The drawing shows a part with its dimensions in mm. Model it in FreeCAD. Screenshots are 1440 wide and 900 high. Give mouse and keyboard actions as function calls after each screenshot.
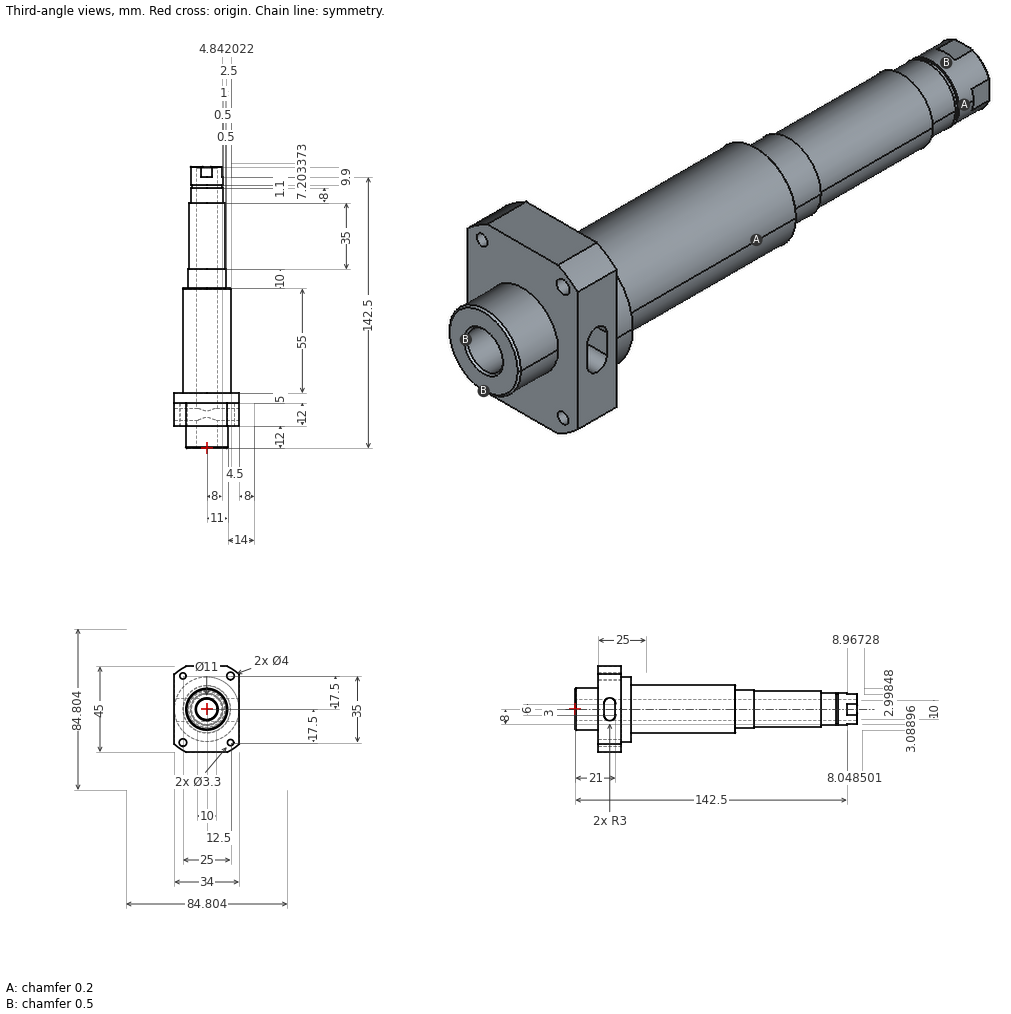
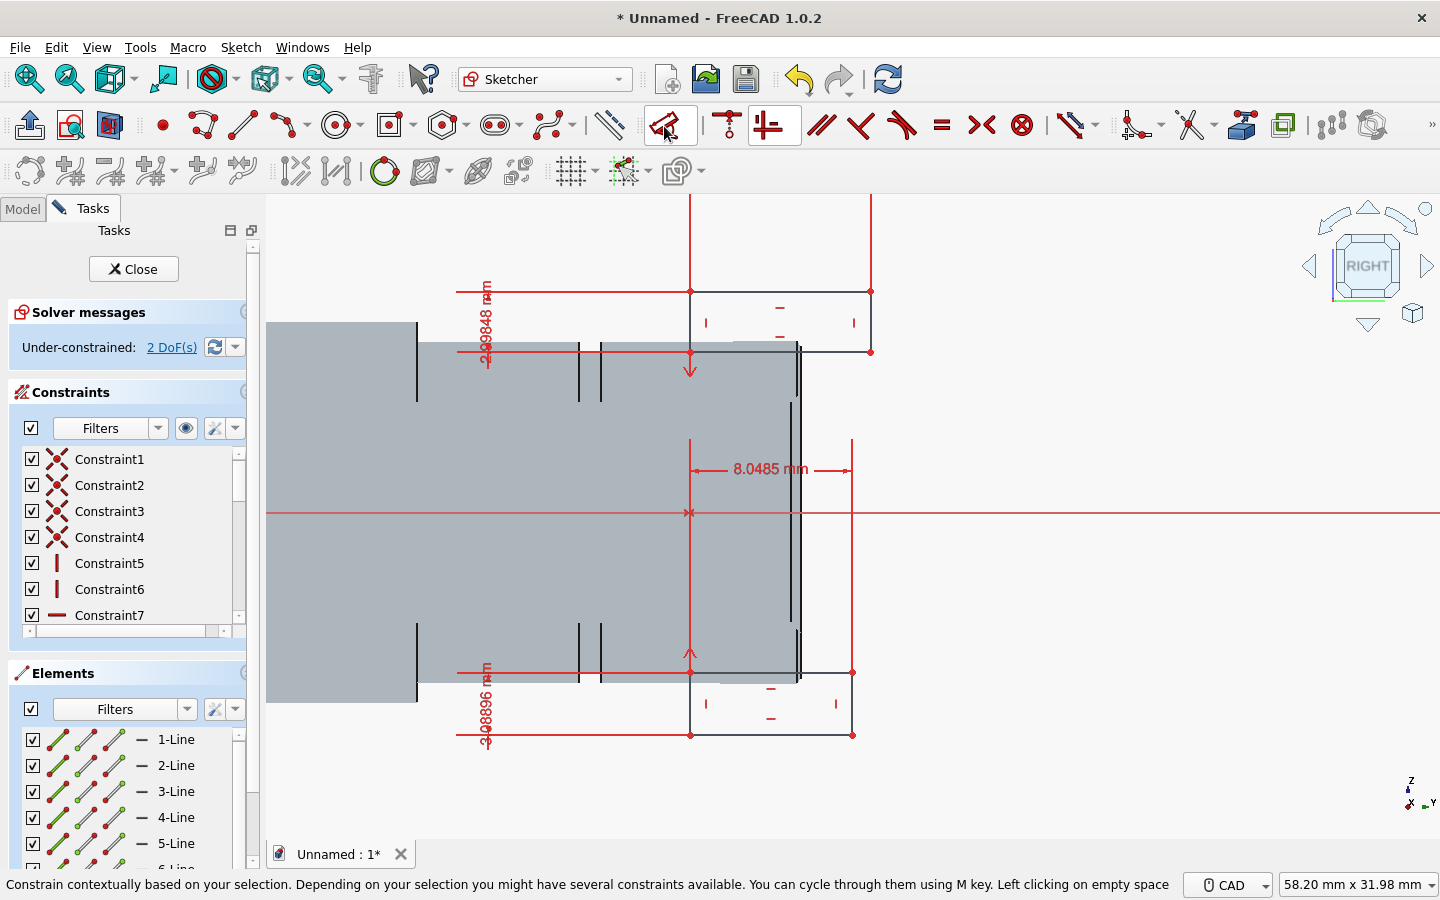
click(690, 673)
click(724, 593)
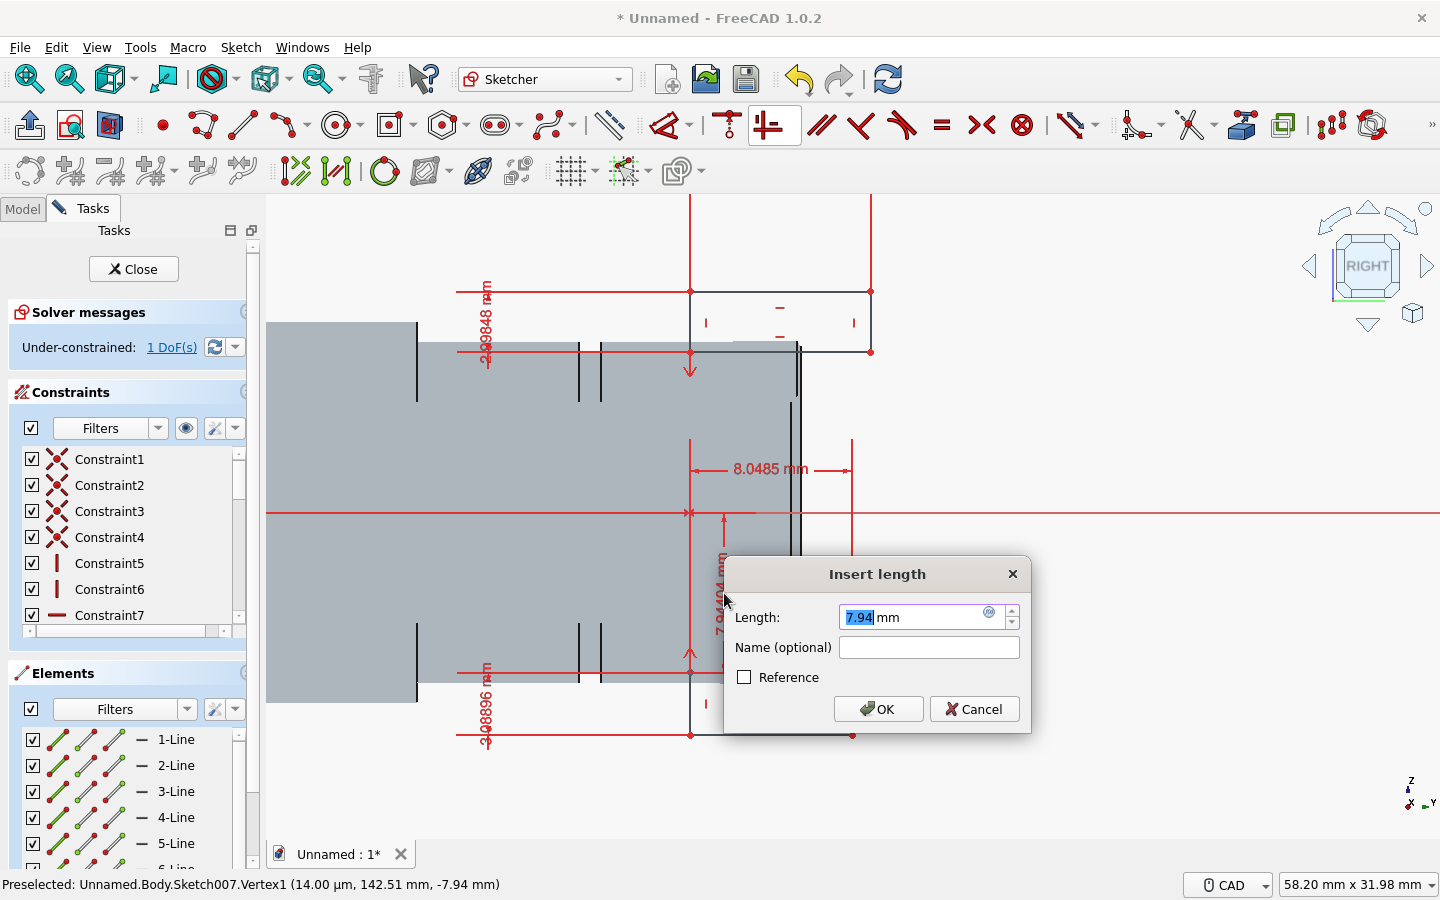
text(8)
key(Return)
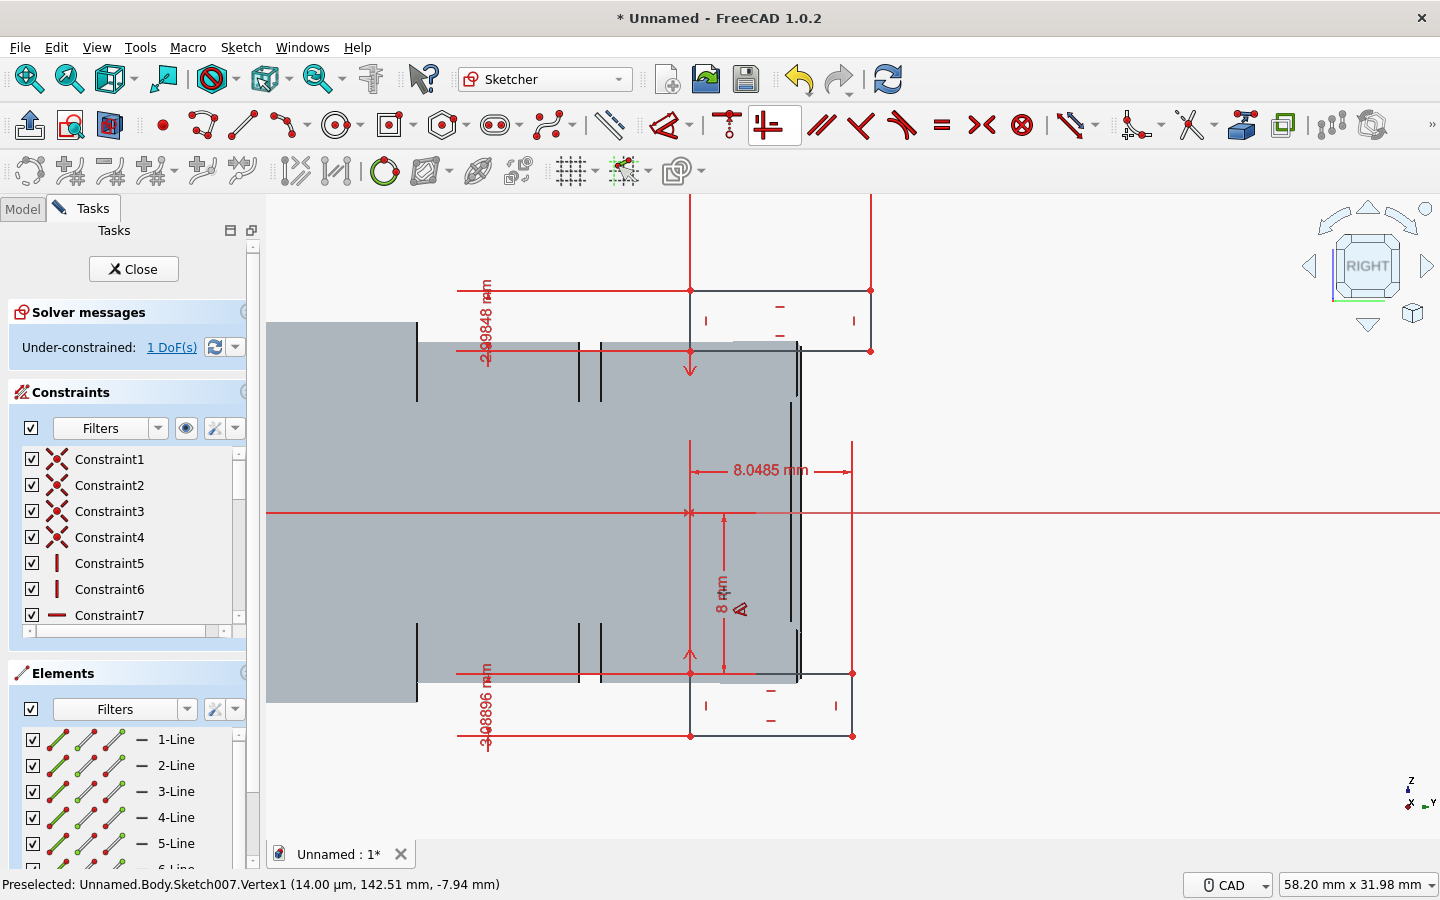
click(690, 674)
click(492, 708)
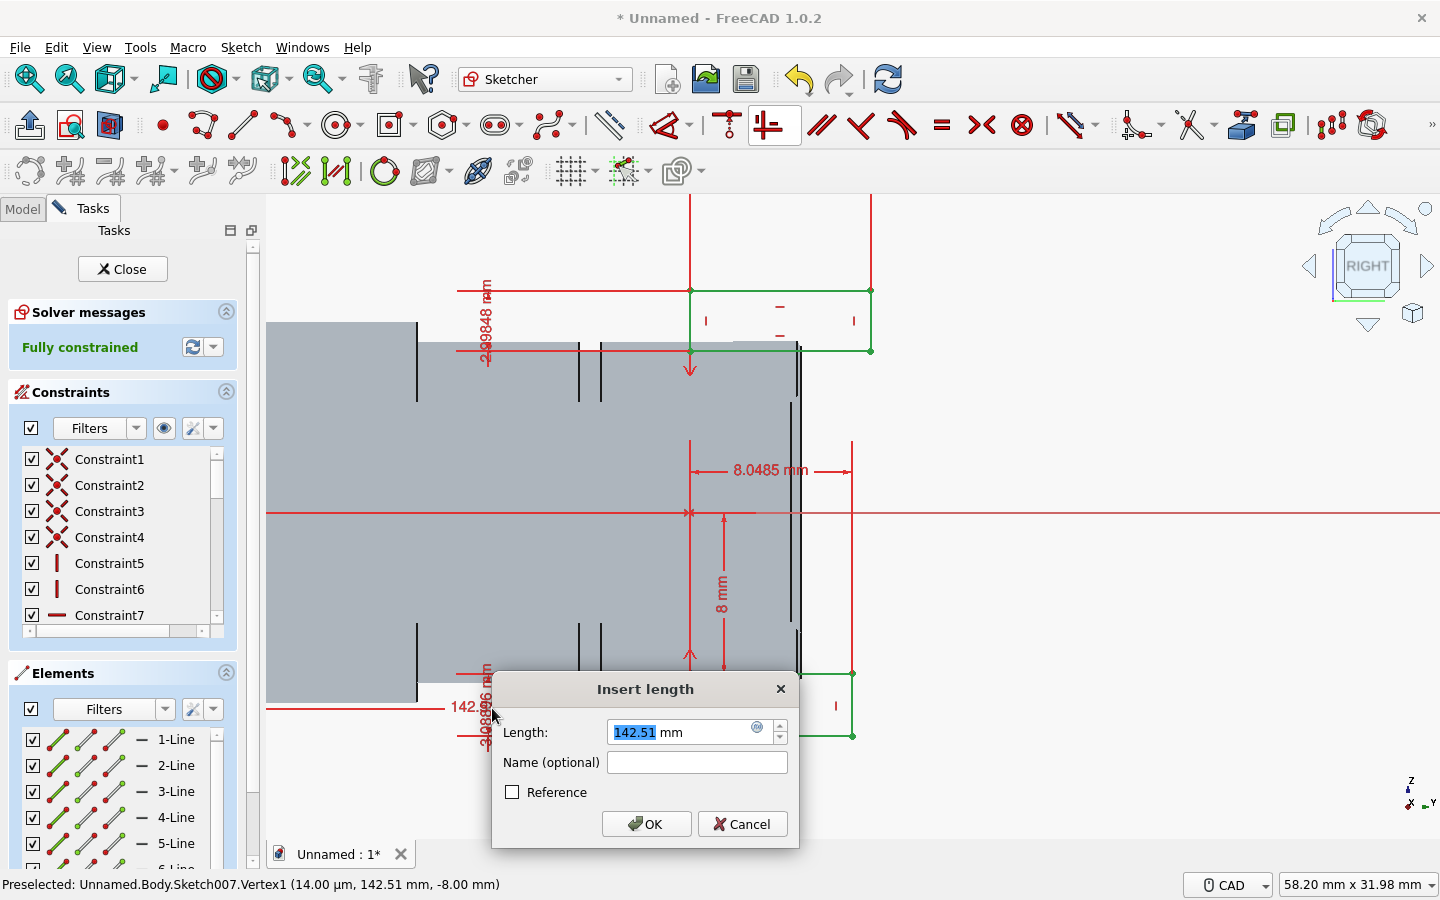
text(142.5)
key(Return)
key(Escape)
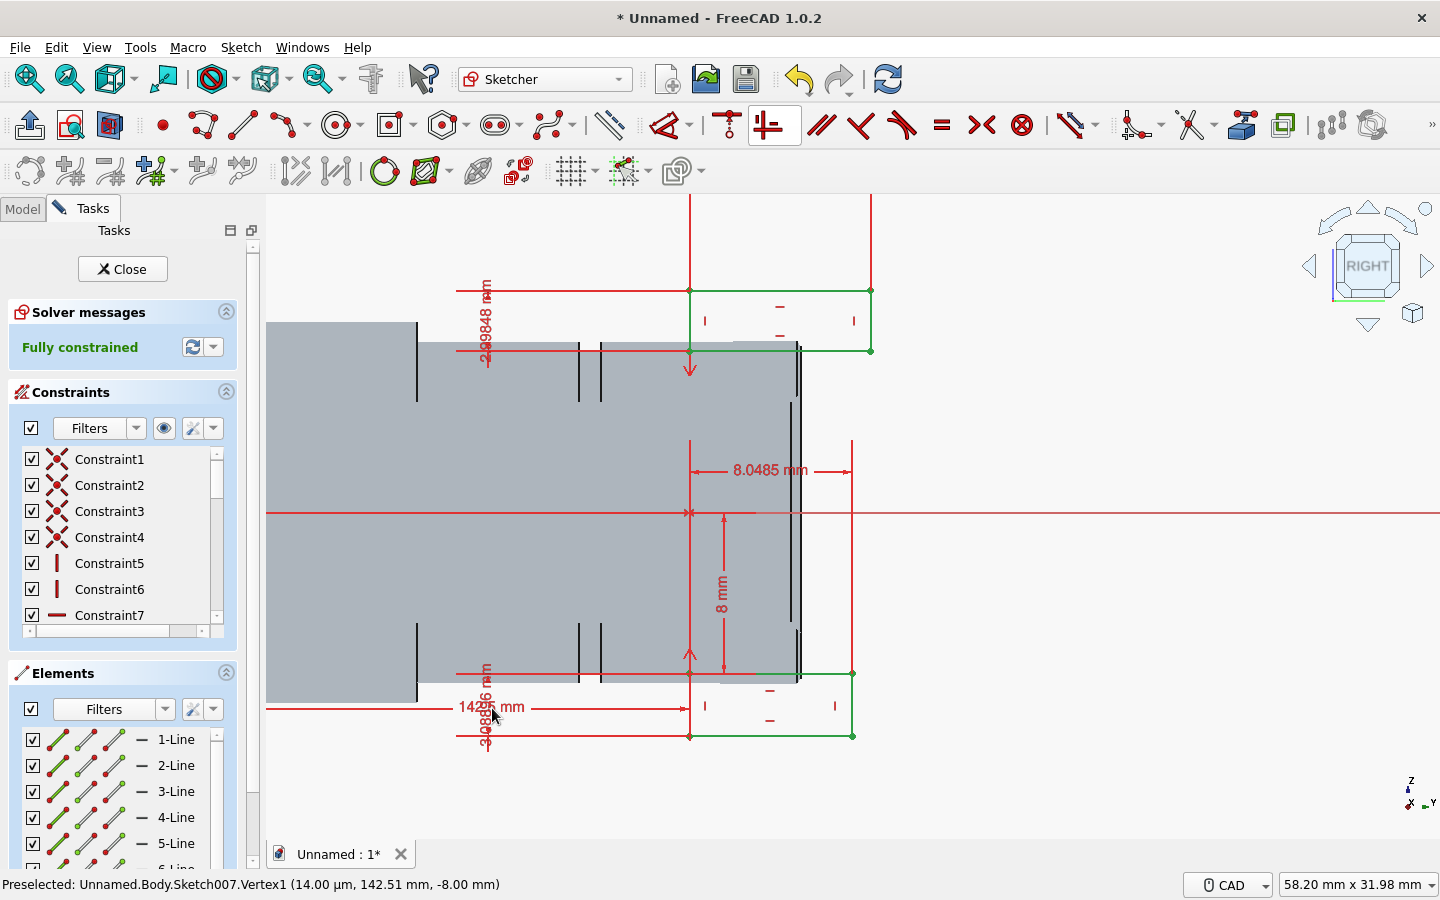
click(123, 269)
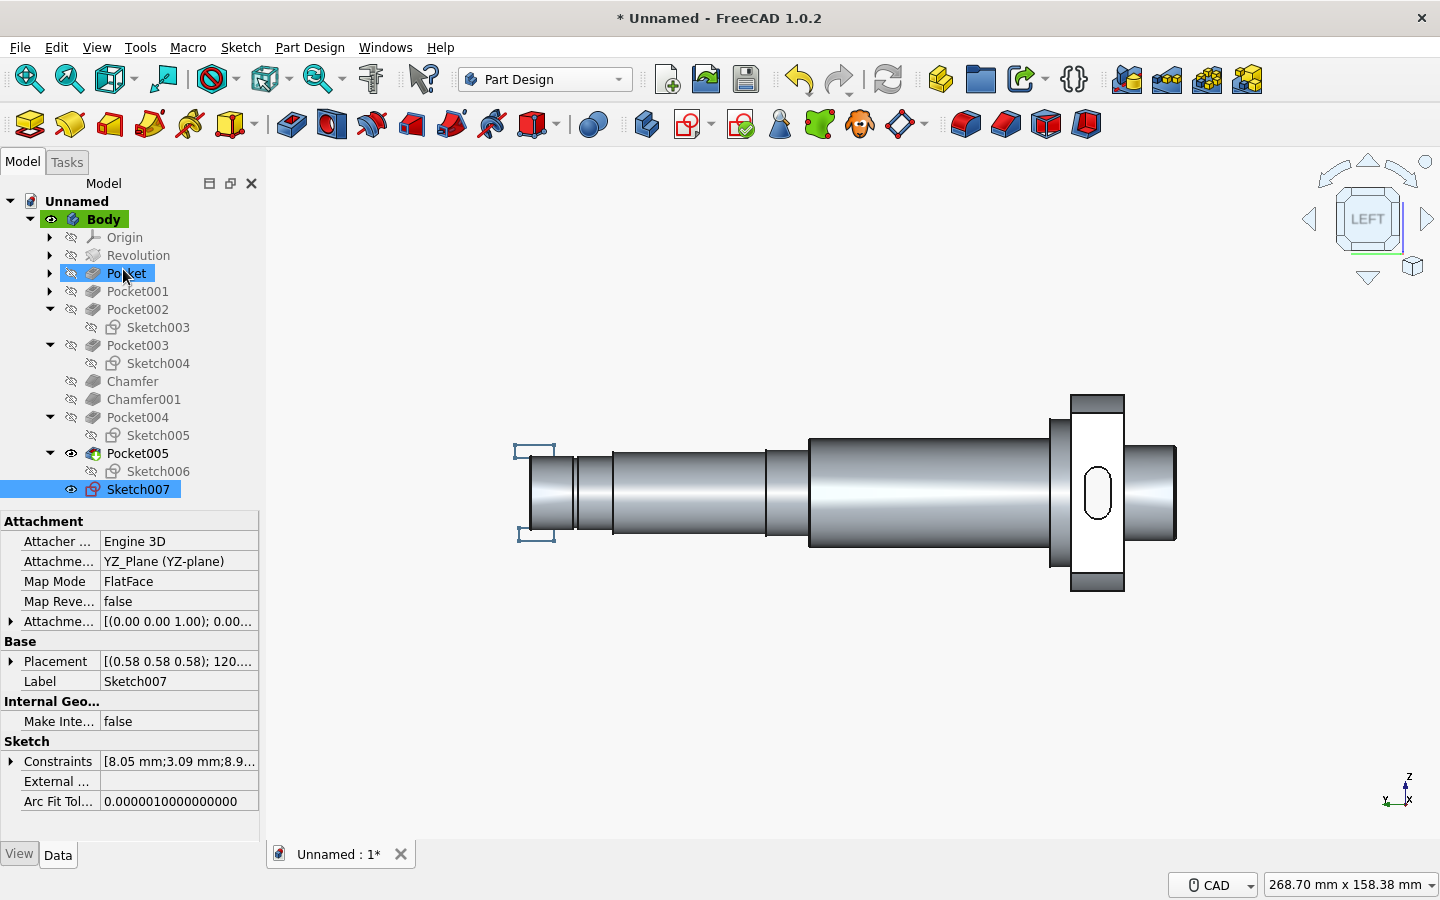
click(292, 124)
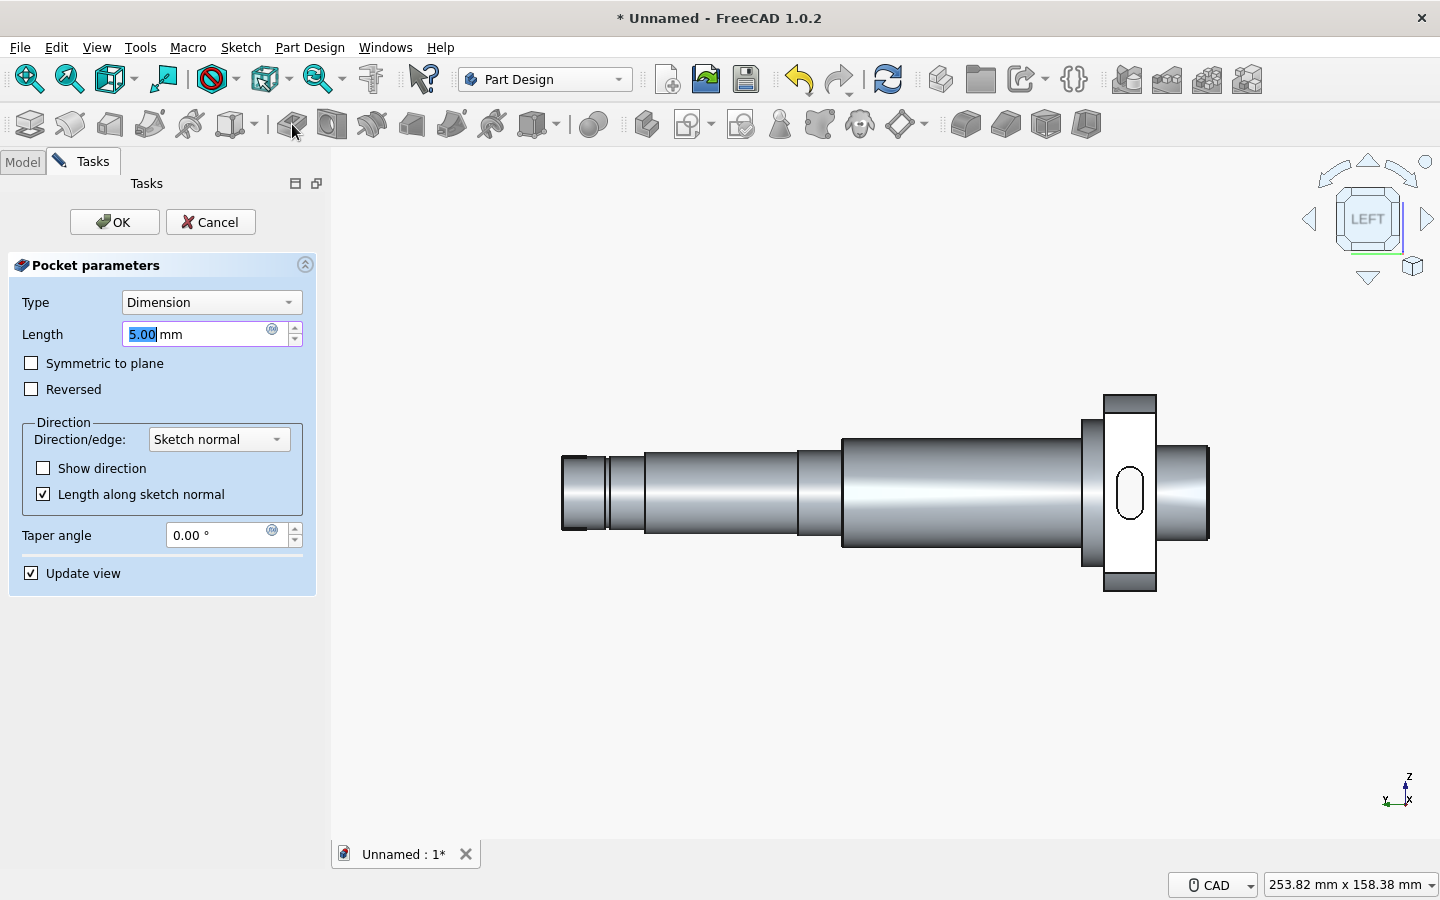
text(10)
key(Tab)